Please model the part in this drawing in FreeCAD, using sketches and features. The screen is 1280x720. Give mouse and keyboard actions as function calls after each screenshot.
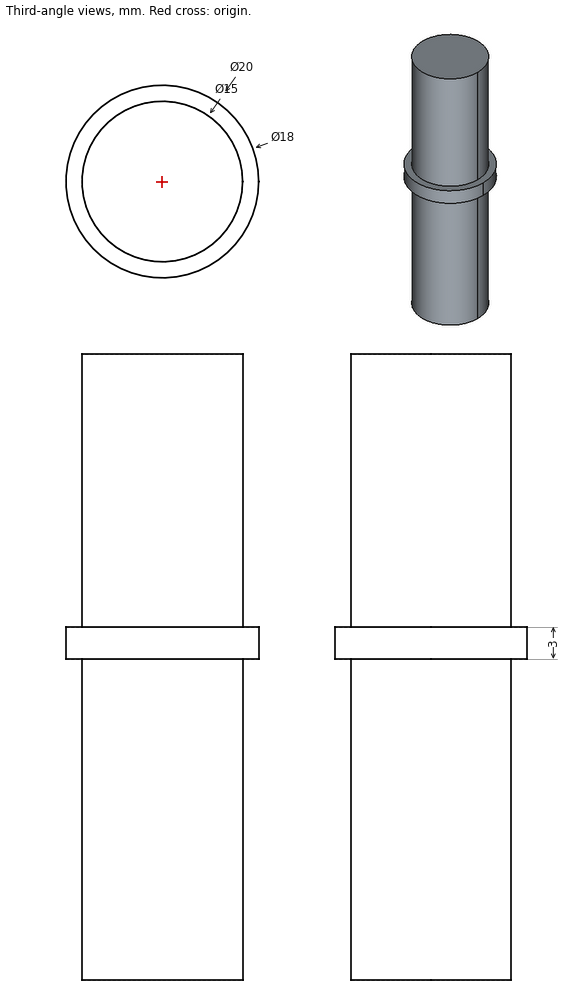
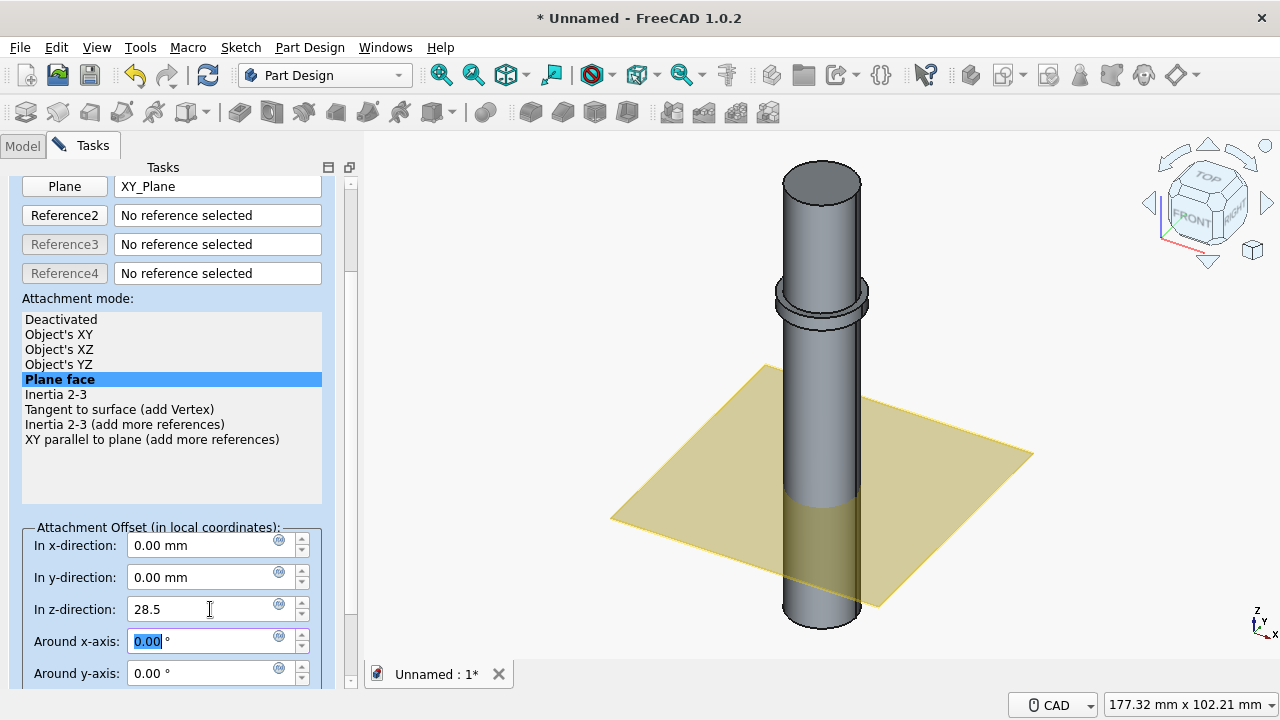
scroll(351, 432, up, 3)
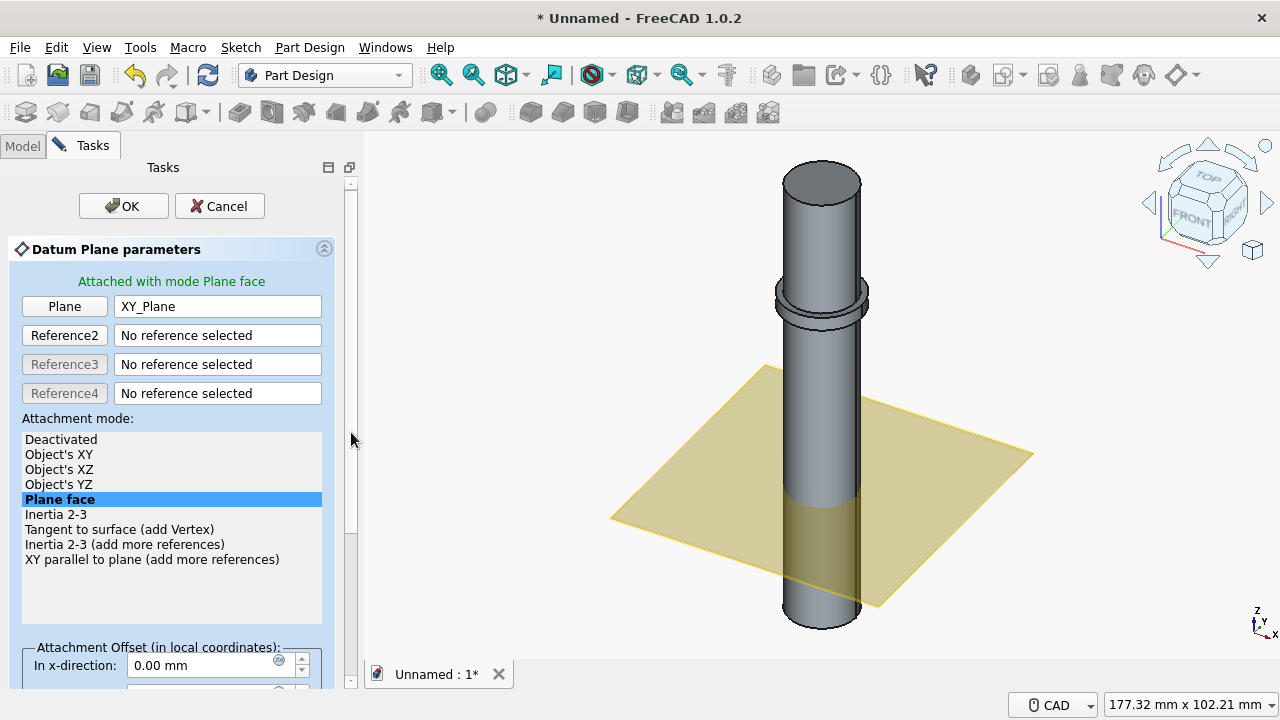
click(124, 206)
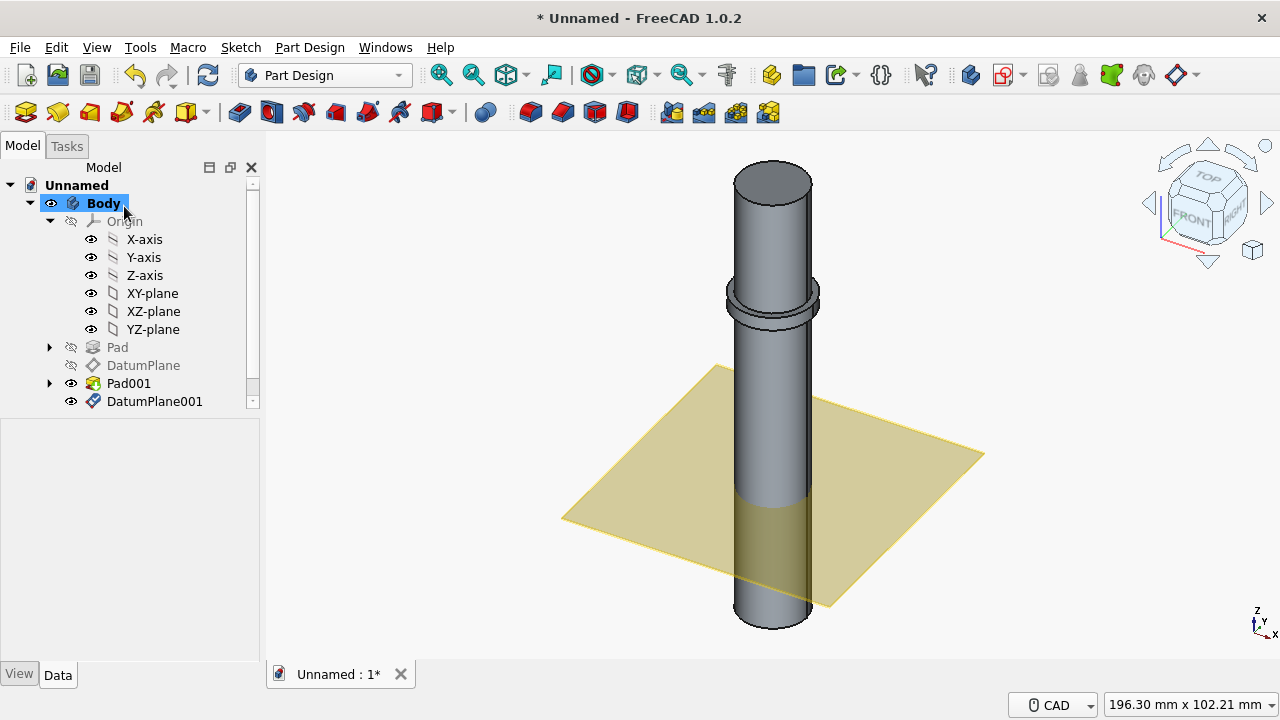
click(116, 401)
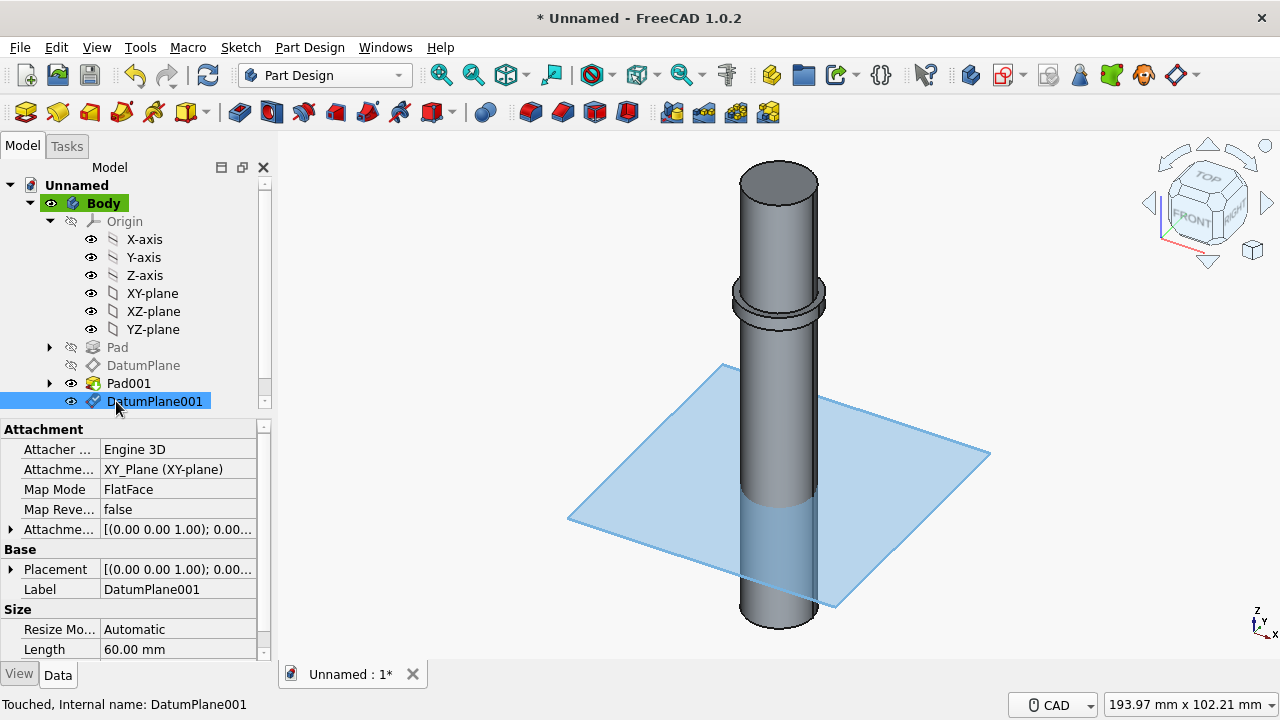
click(1004, 76)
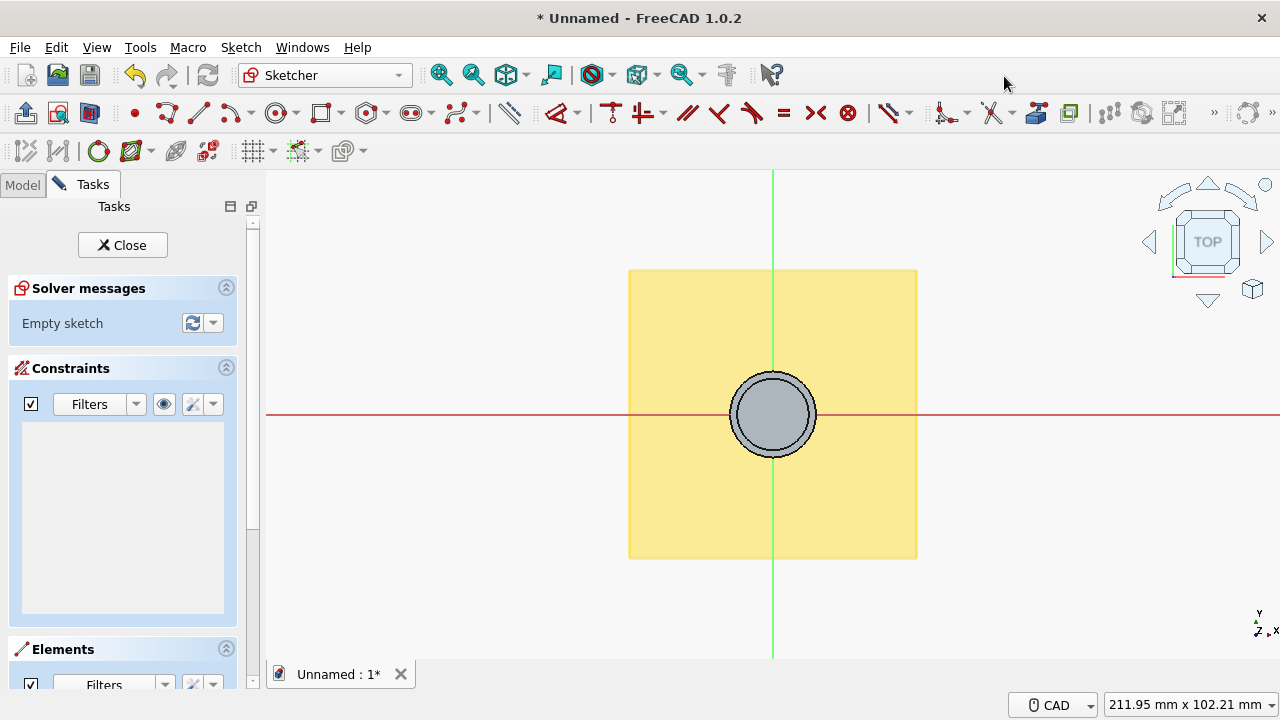
key(q)
key(s)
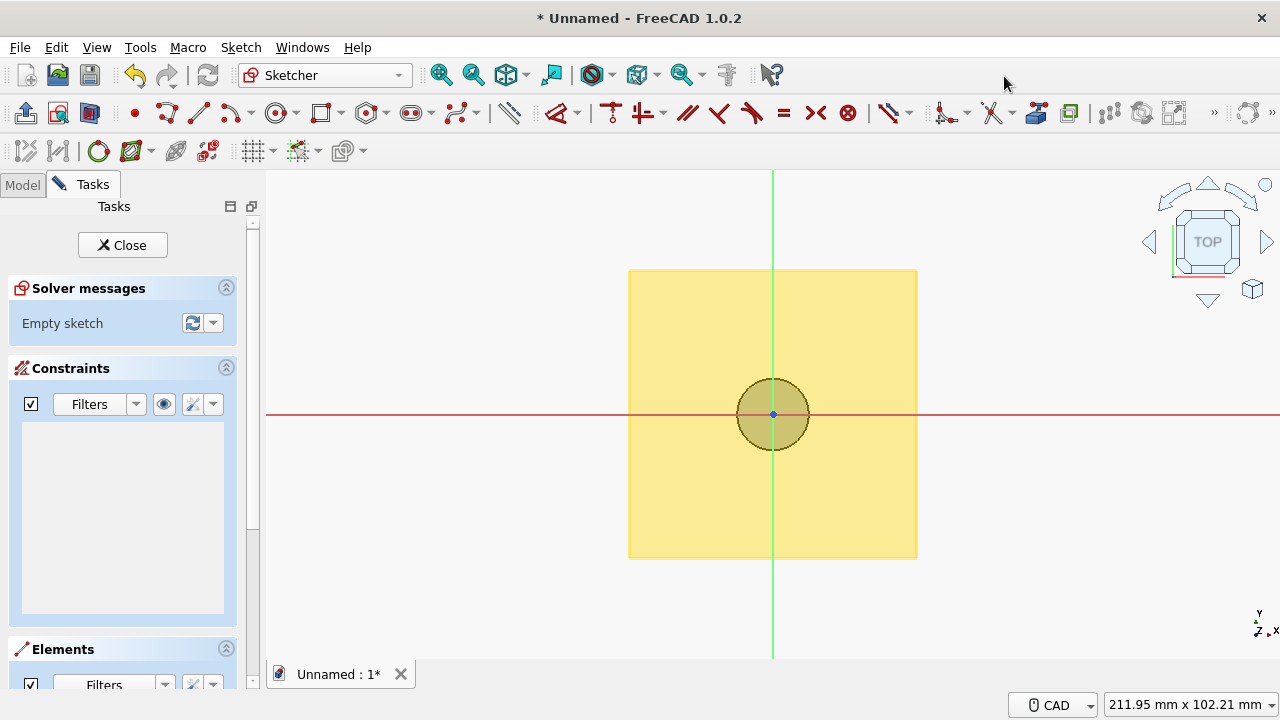
scroll(803, 415, up, 6)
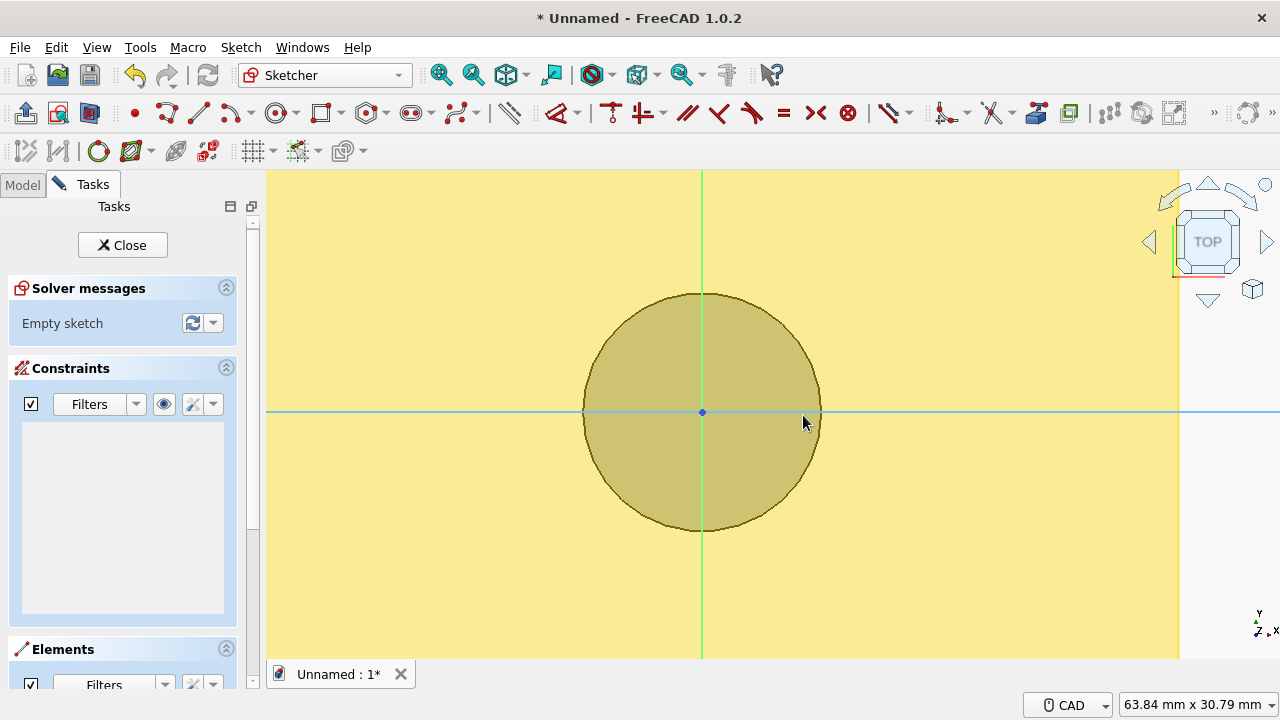
click(276, 114)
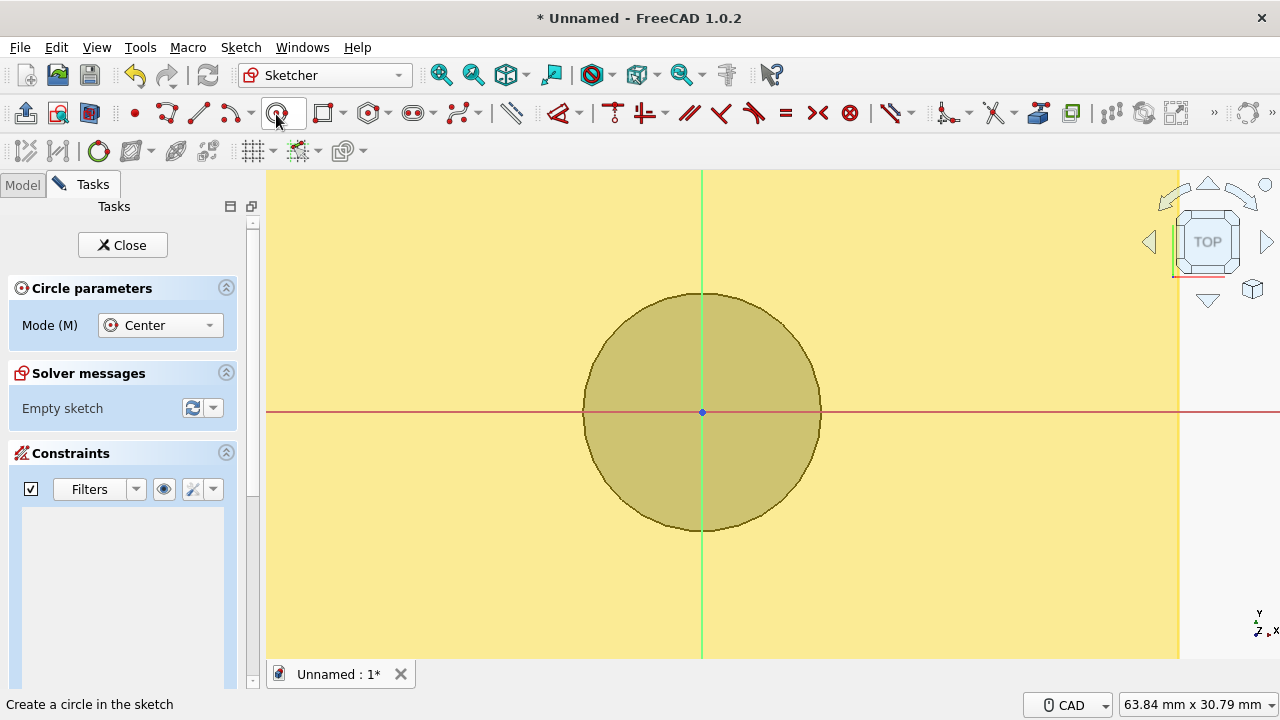
click(702, 412)
click(803, 311)
key(Escape)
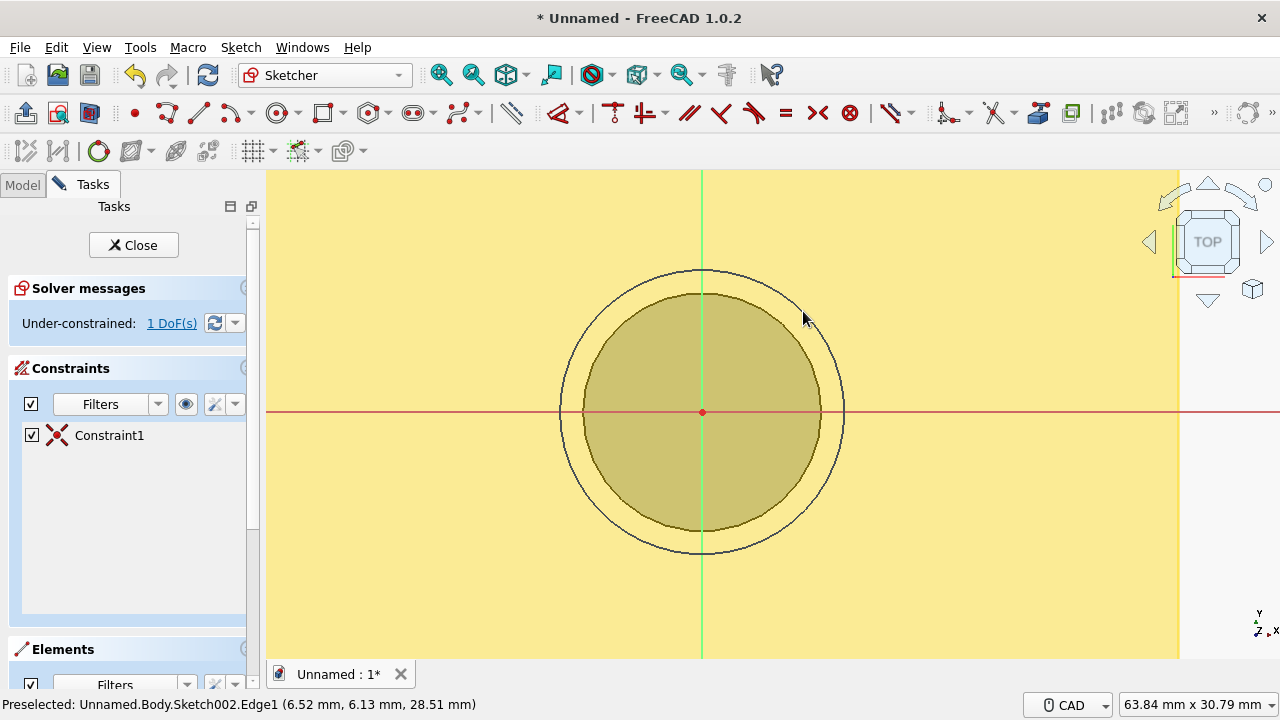
click(558, 114)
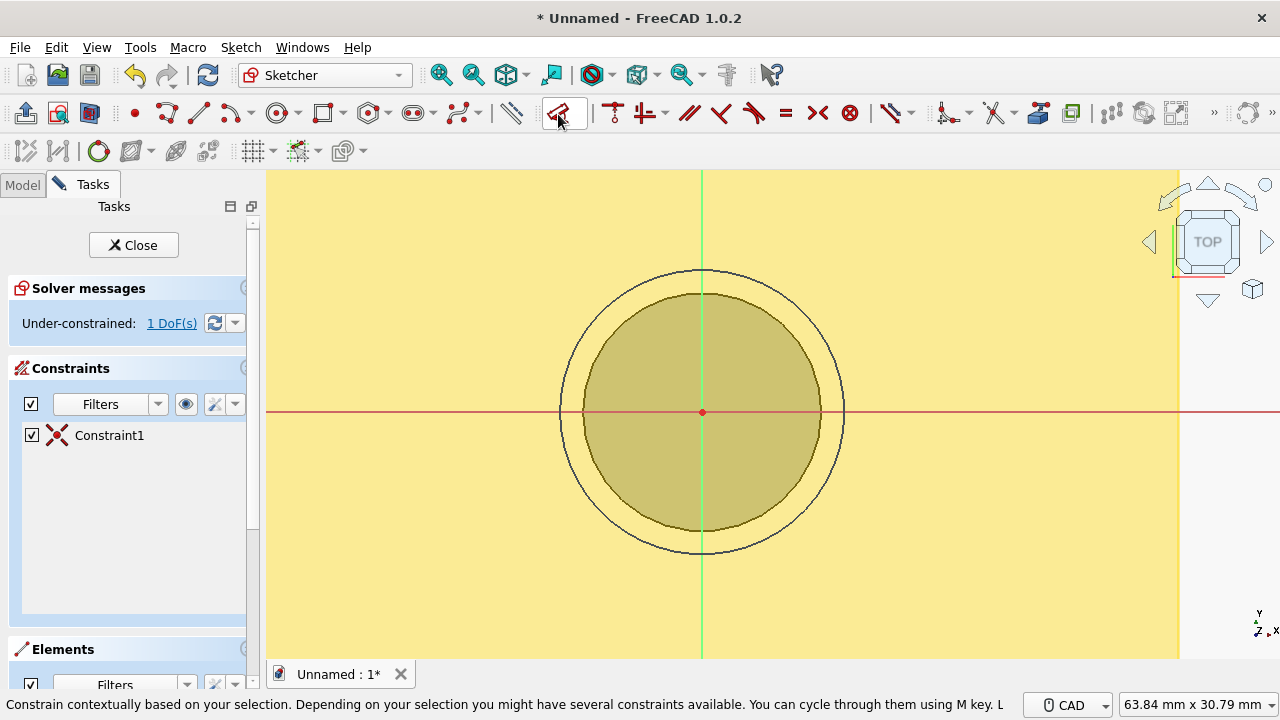
click(802, 311)
click(824, 288)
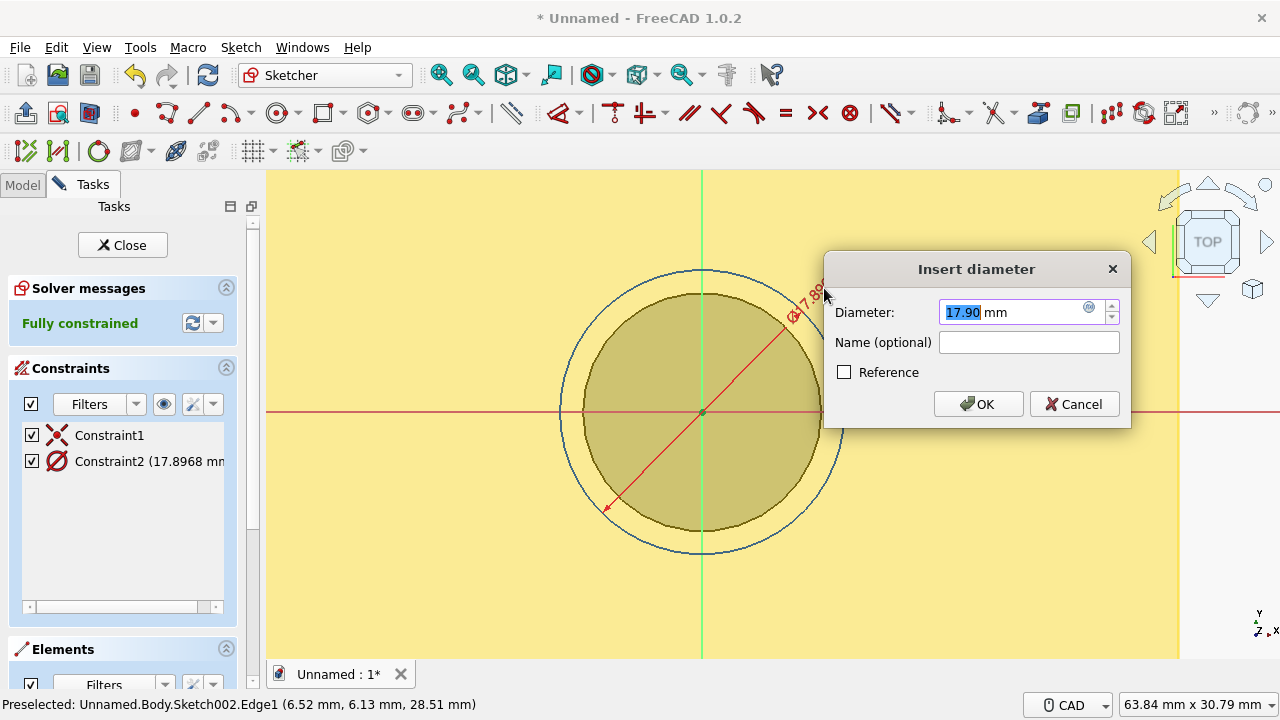
text(18)
key(Return)
key(Escape)